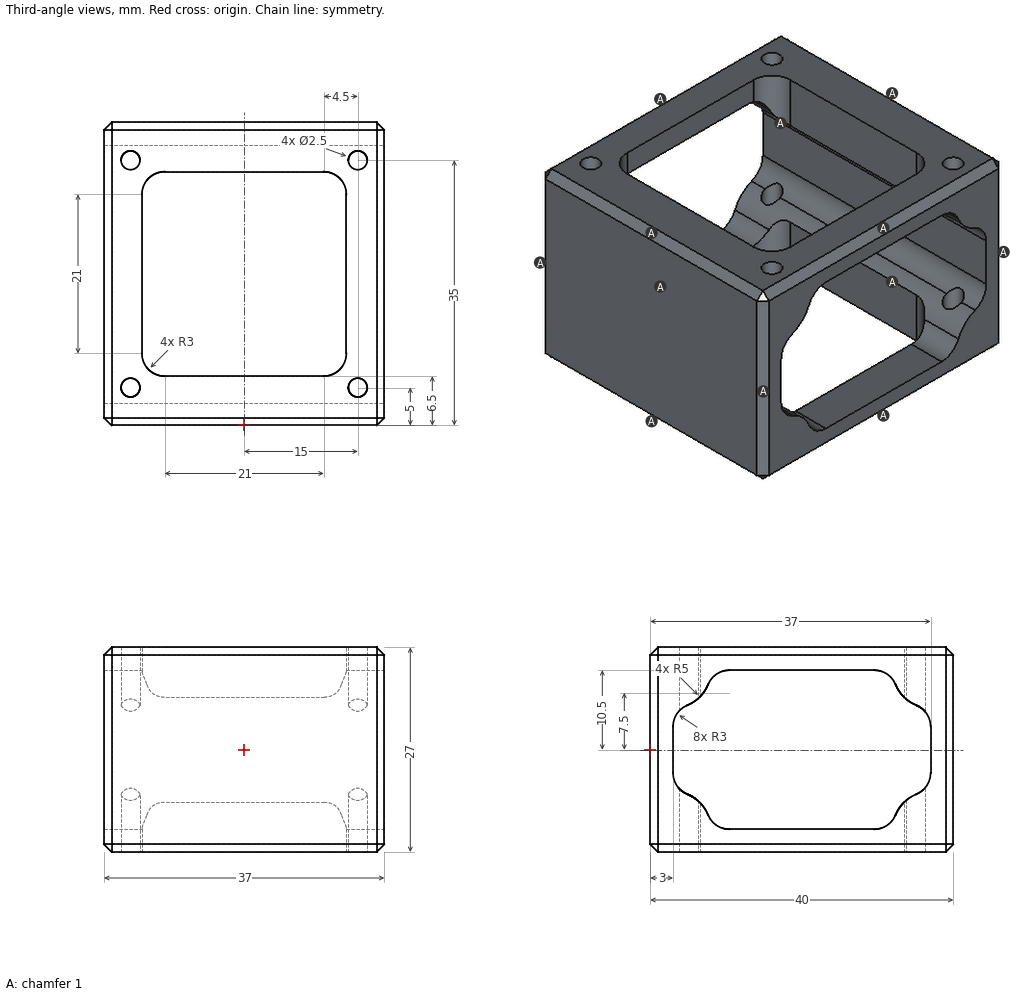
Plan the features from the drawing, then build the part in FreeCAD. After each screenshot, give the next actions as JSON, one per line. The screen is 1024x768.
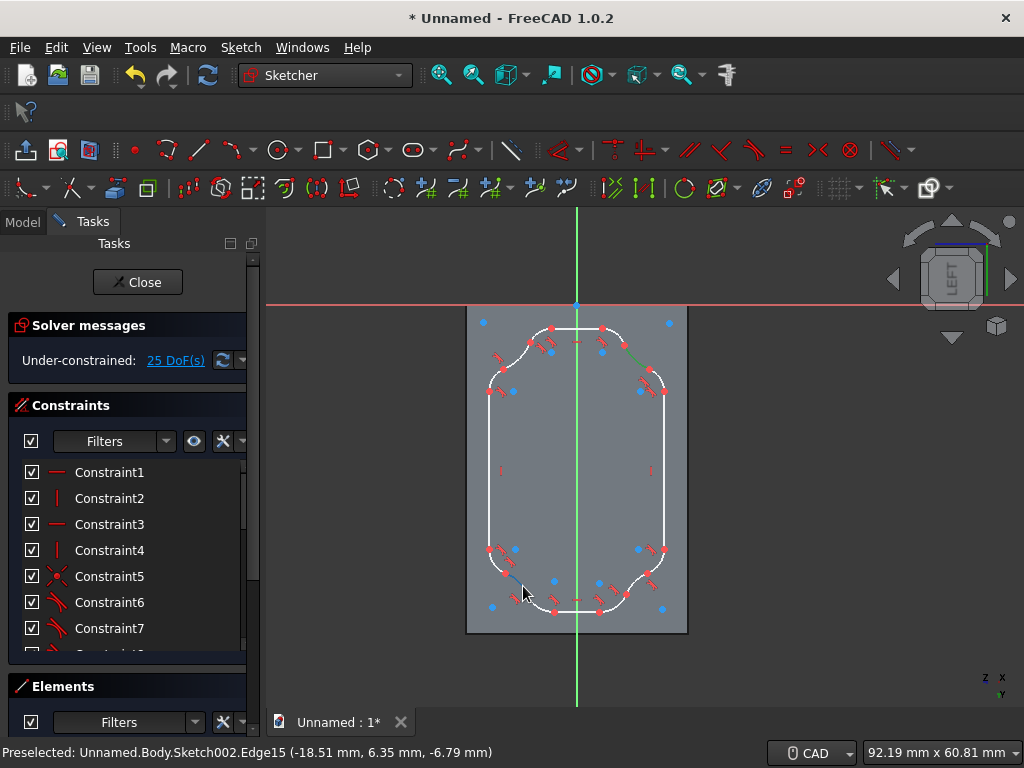
{"action": "scroll", "coordinate": [621, 338], "scroll_direction": "up", "scroll_amount": 3}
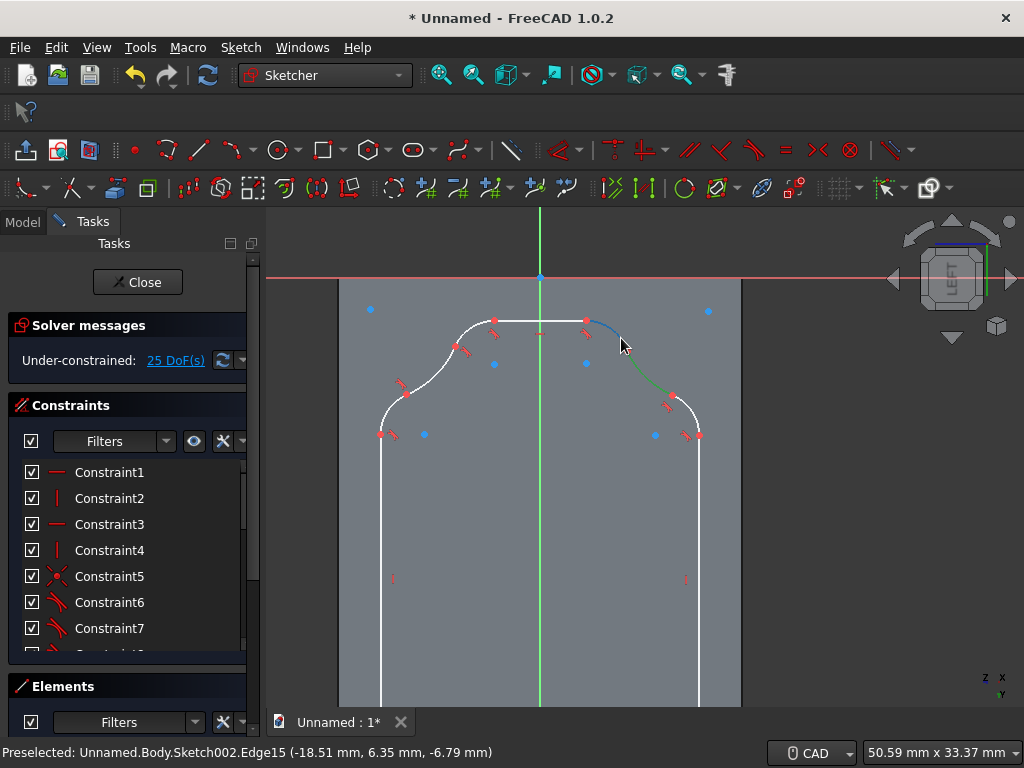
{"action": "left_click", "coordinate": [620, 337]}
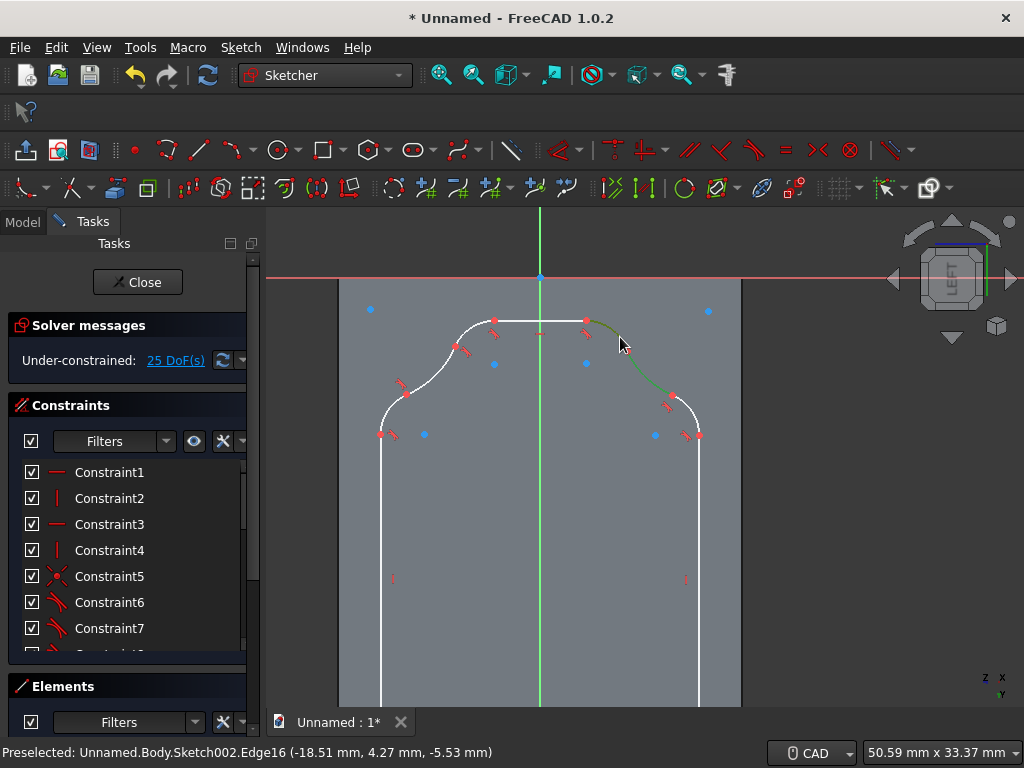
{"action": "key", "text": "t"}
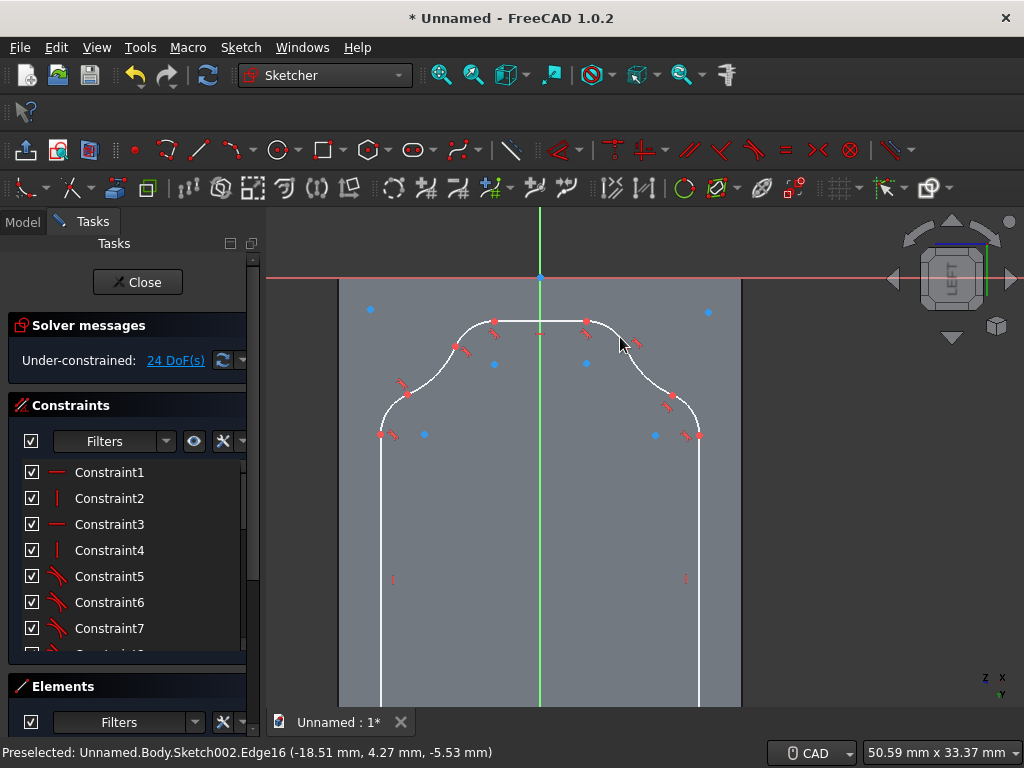
{"action": "left_click", "coordinate": [480, 324]}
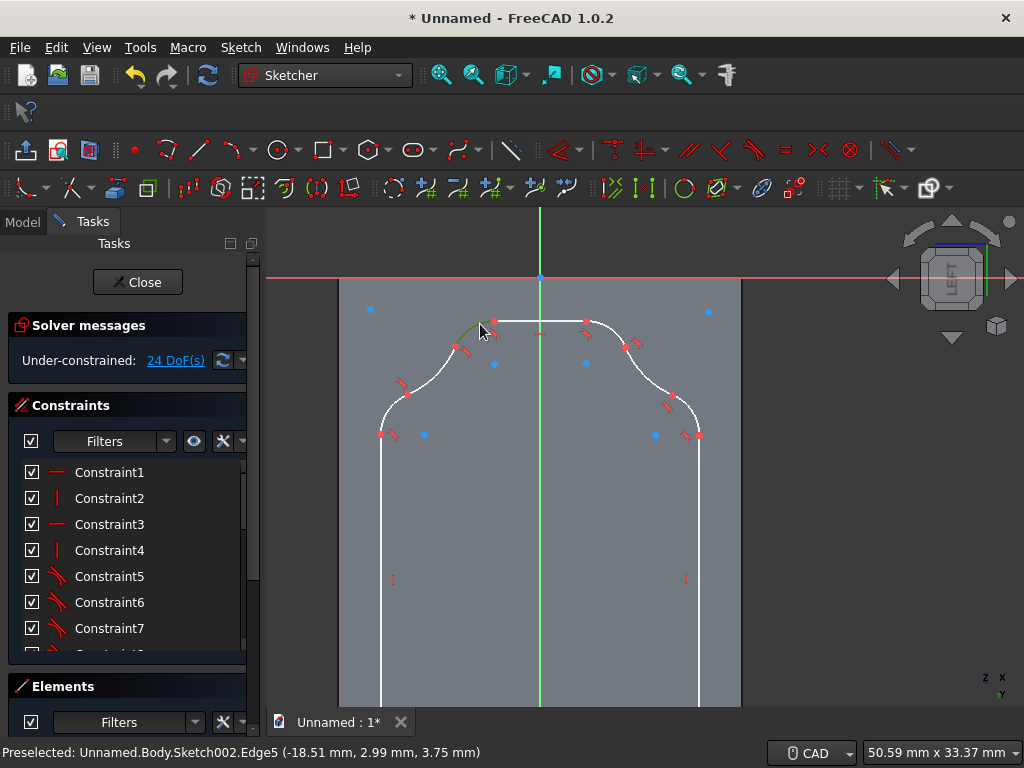
{"action": "left_click", "coordinate": [394, 403]}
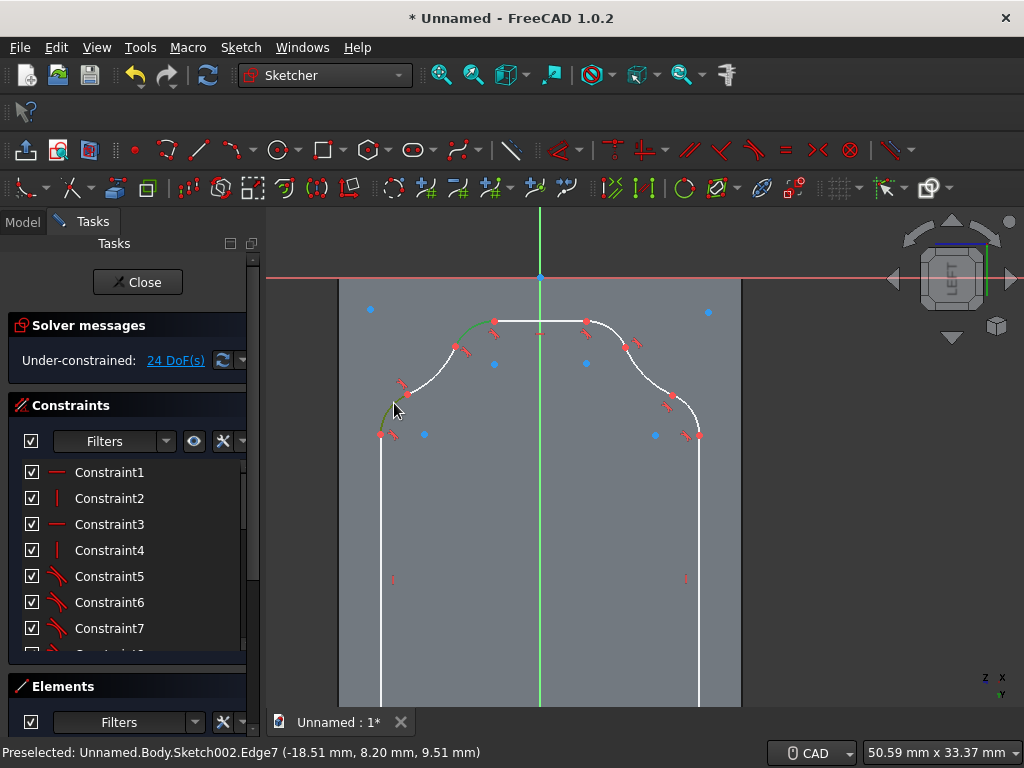
{"action": "scroll", "coordinate": [621, 338], "scroll_direction": "down", "scroll_amount": 3}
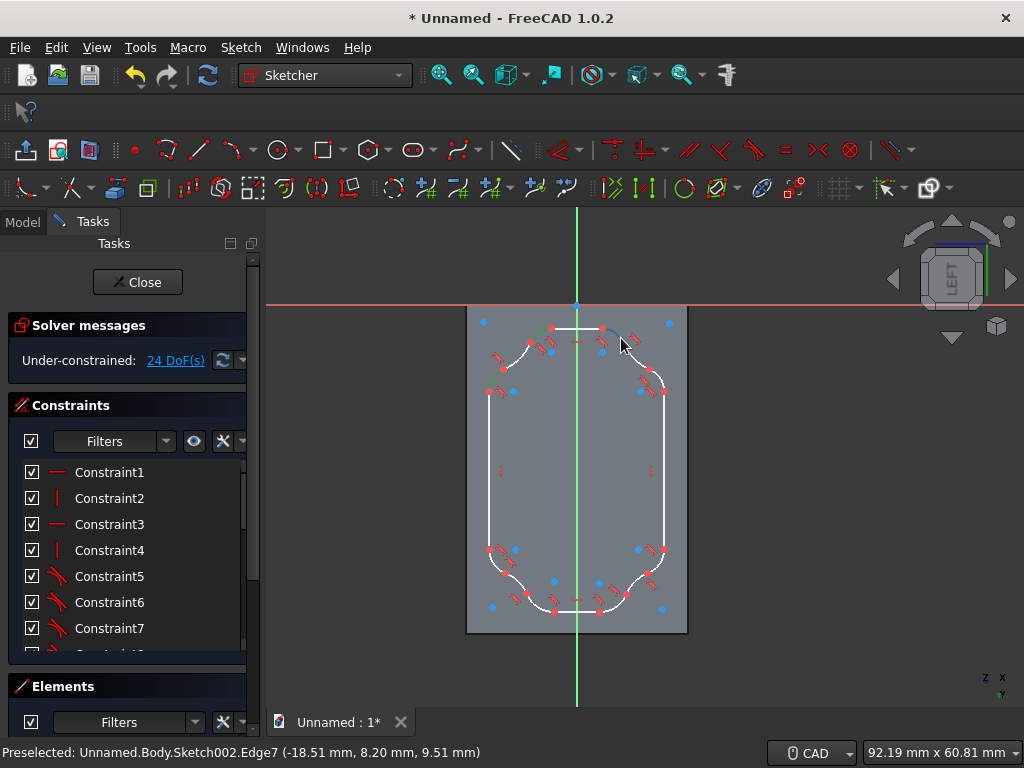
{"action": "scroll", "coordinate": [491, 559], "scroll_direction": "up", "scroll_amount": 3}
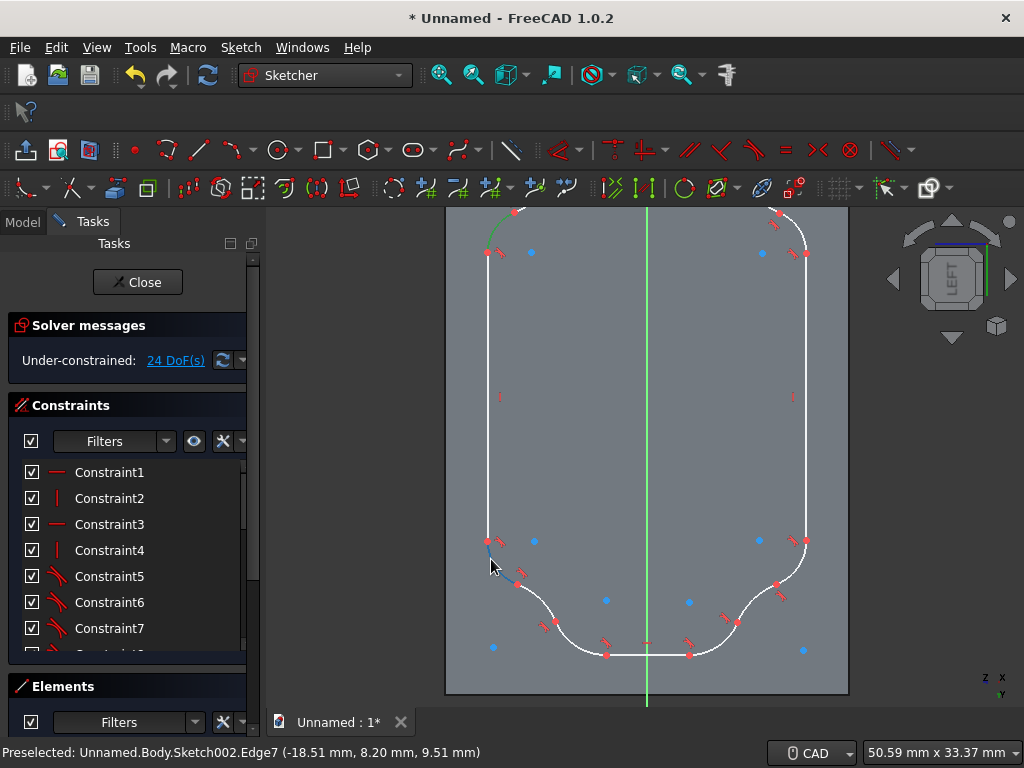
{"action": "left_click", "coordinate": [491, 558]}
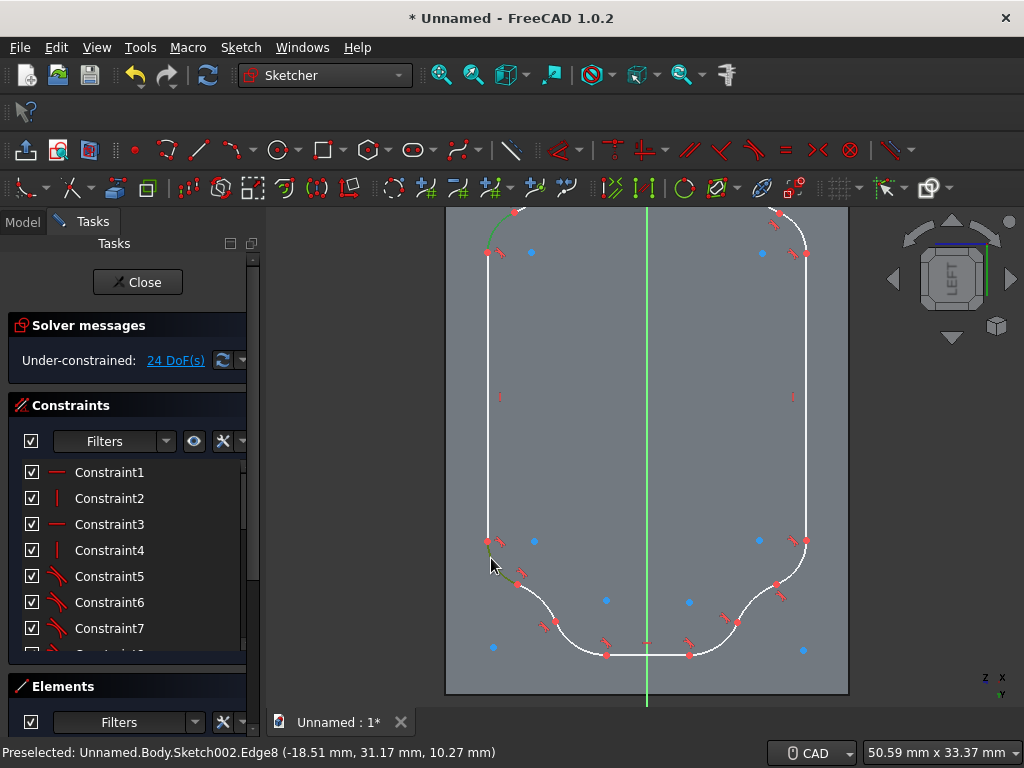
{"action": "left_click", "coordinate": [566, 638]}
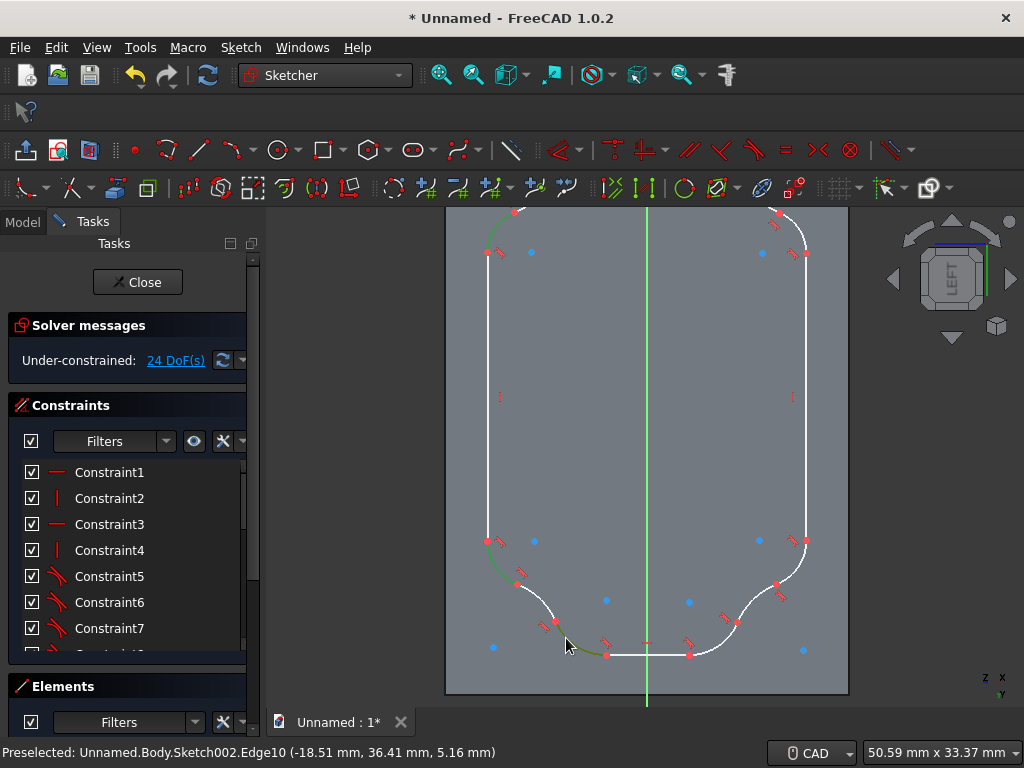
{"action": "left_click", "coordinate": [707, 652]}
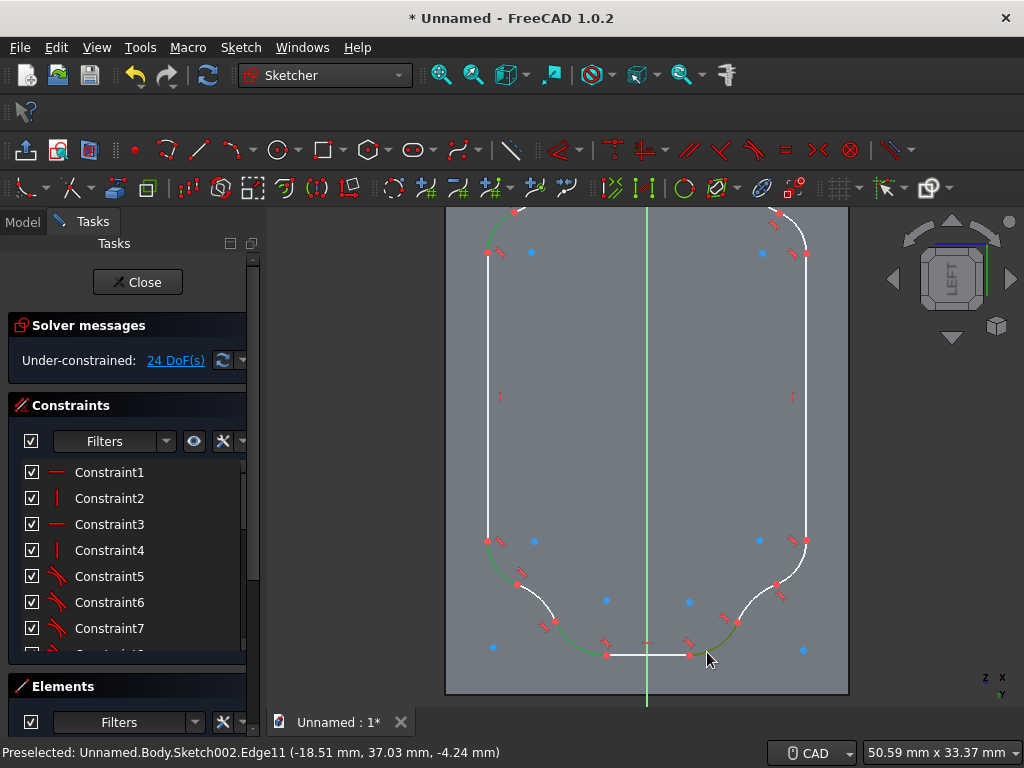
{"action": "left_click", "coordinate": [791, 575]}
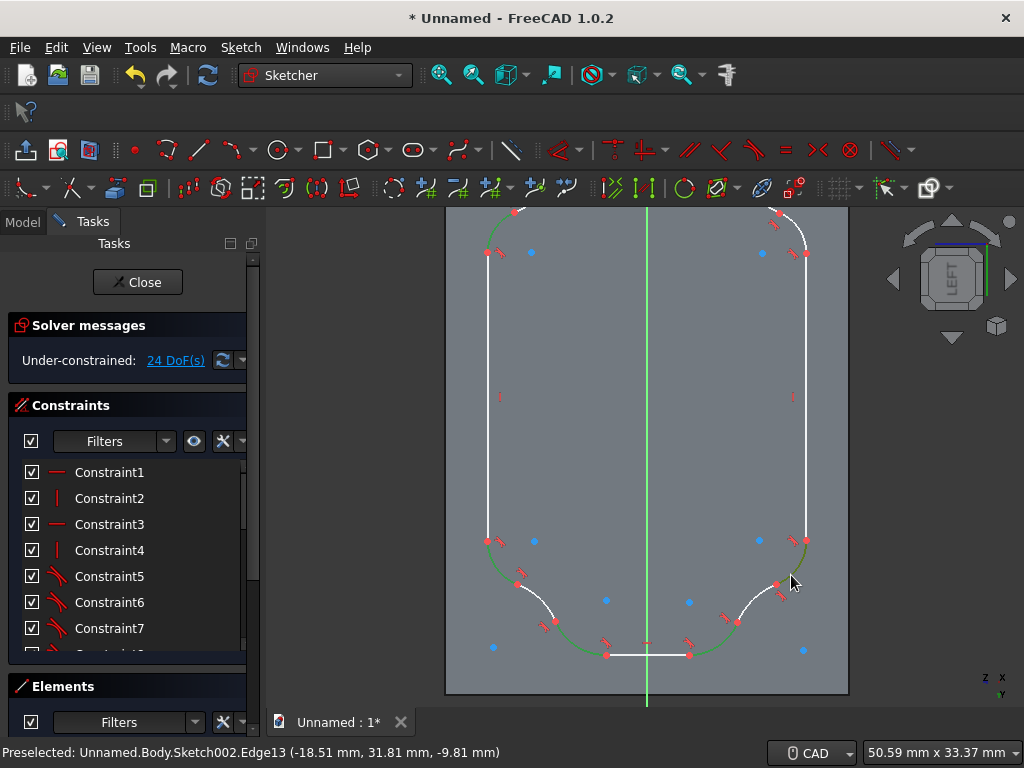
{"action": "left_click", "coordinate": [804, 238]}